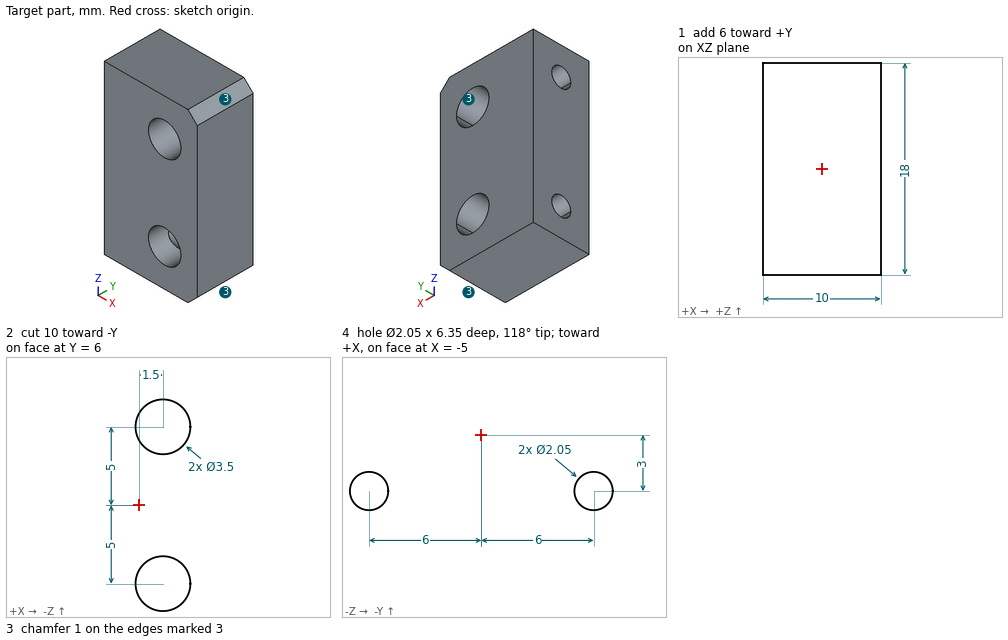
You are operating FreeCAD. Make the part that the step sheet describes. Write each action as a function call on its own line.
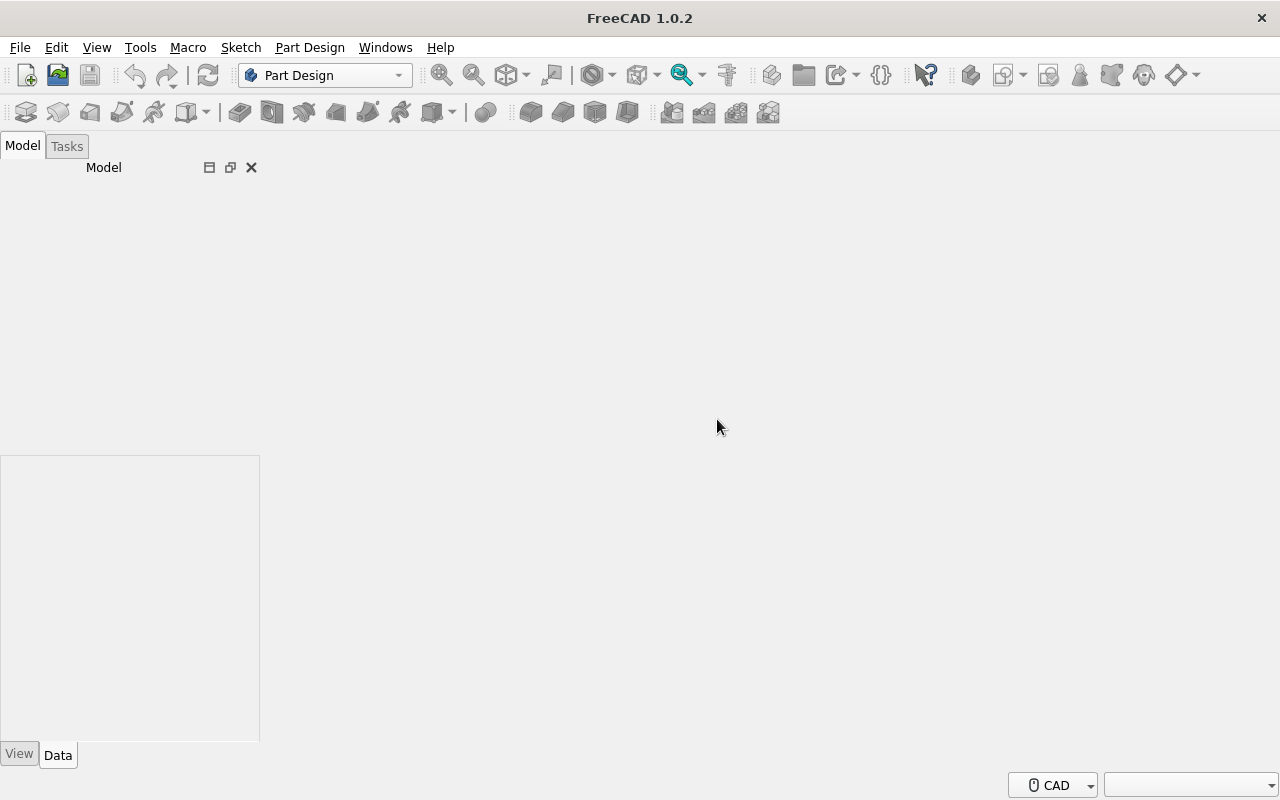
key(ctrl+n)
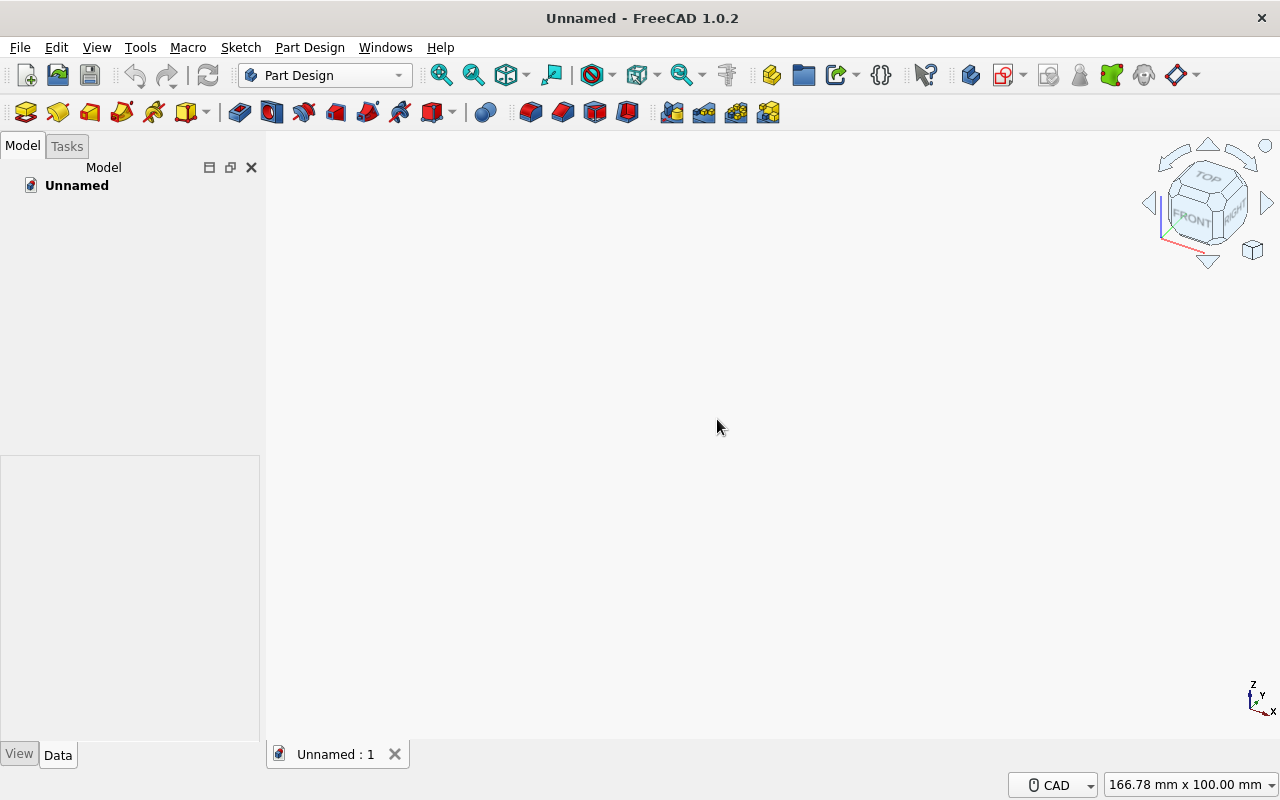
click(1004, 76)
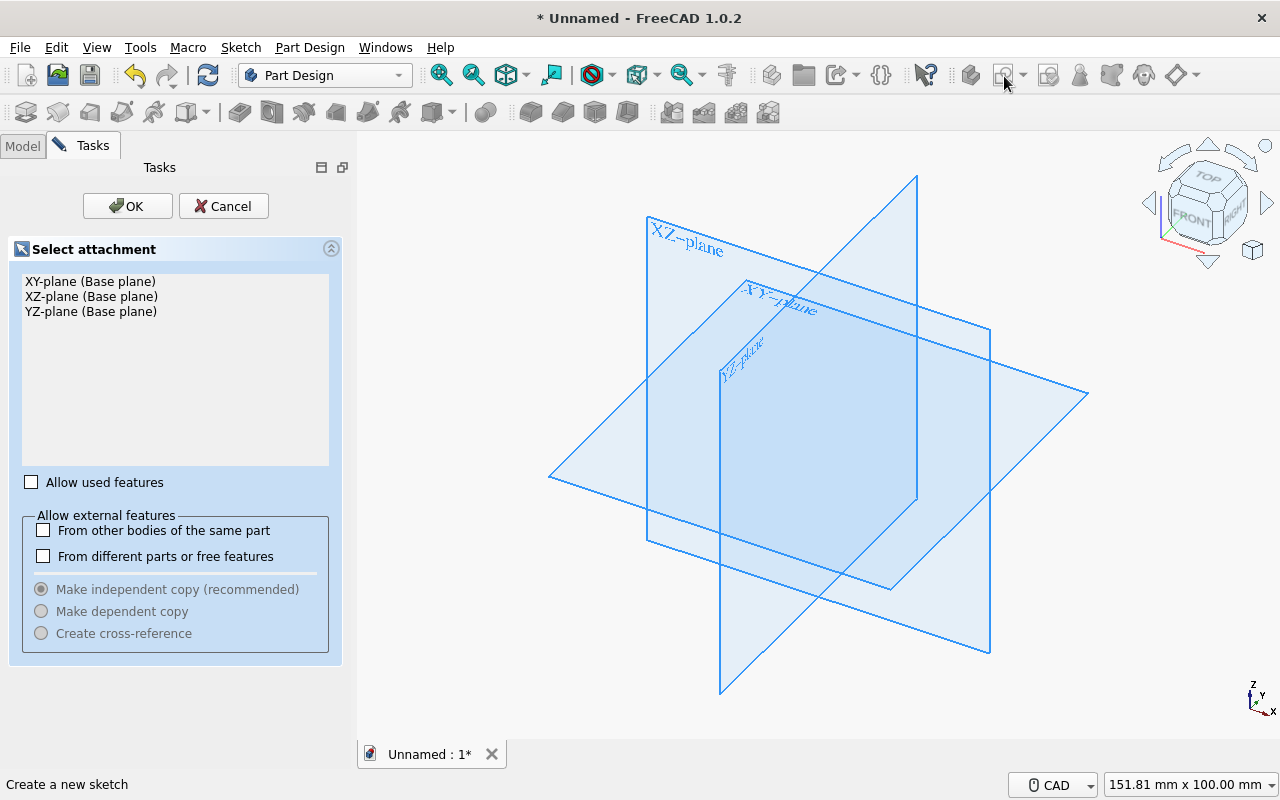
click(82, 296)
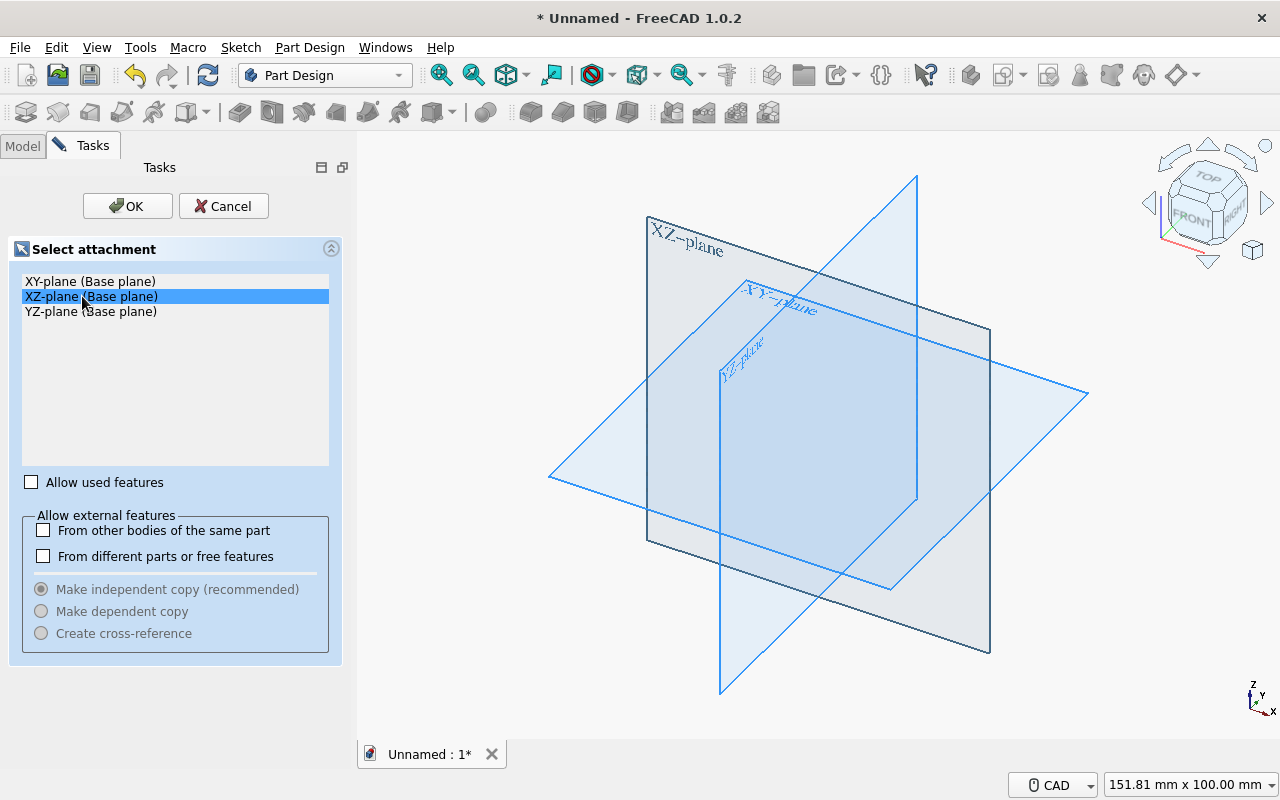
click(128, 206)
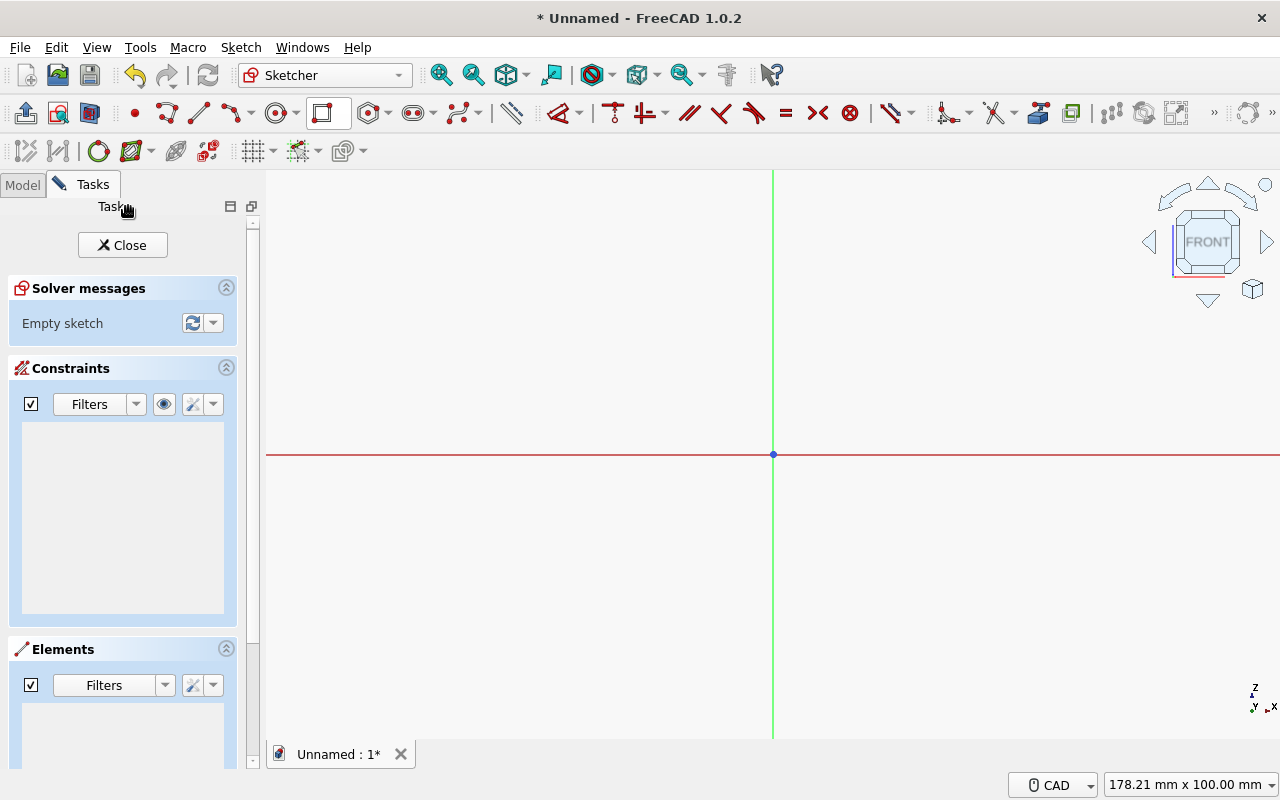
scroll(803, 455, up, 6)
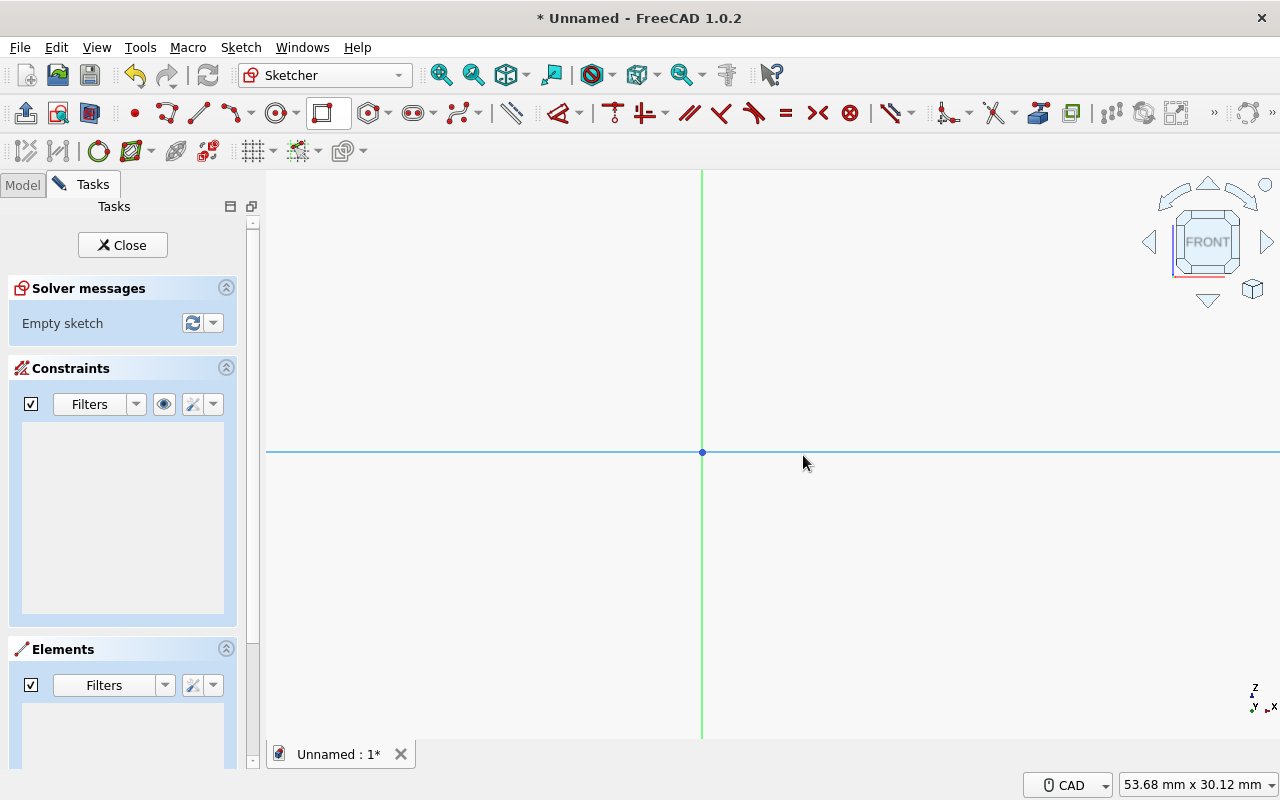
key(g)
key(v)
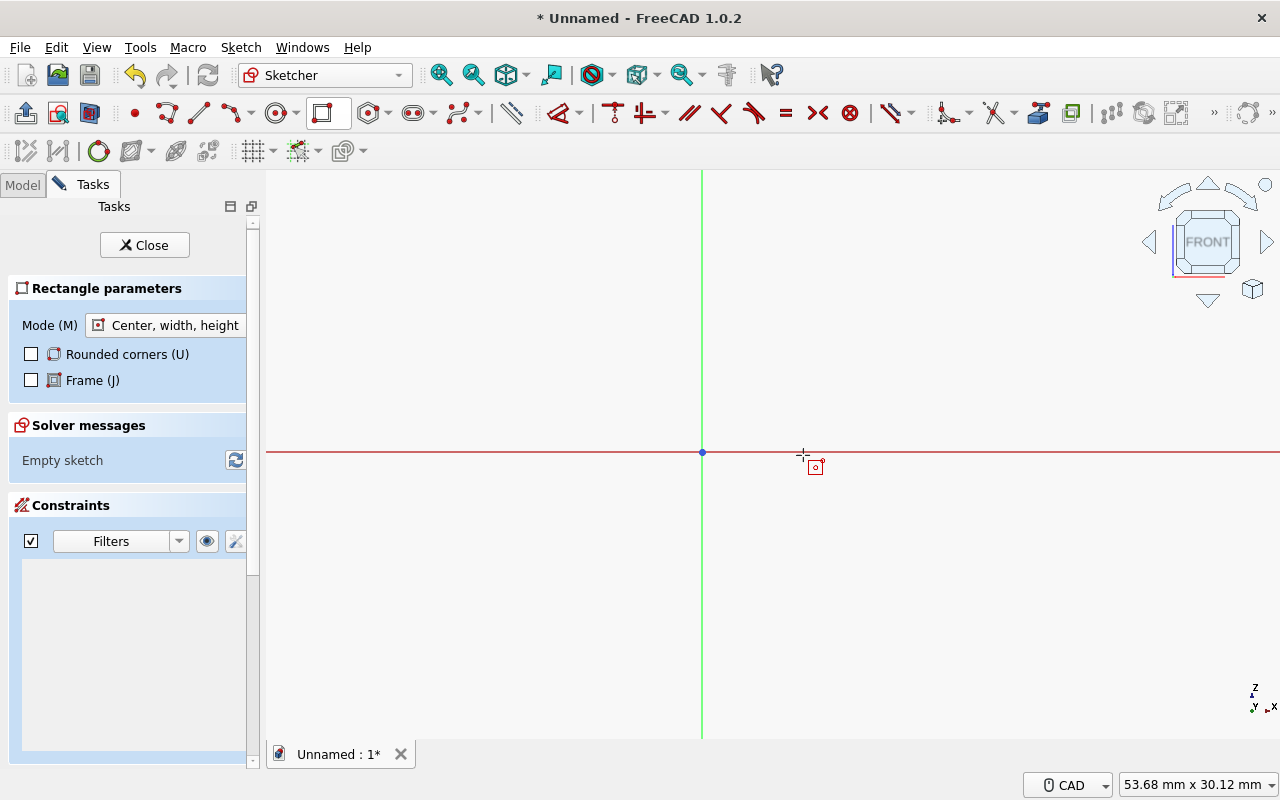
click(702, 452)
move(797, 282)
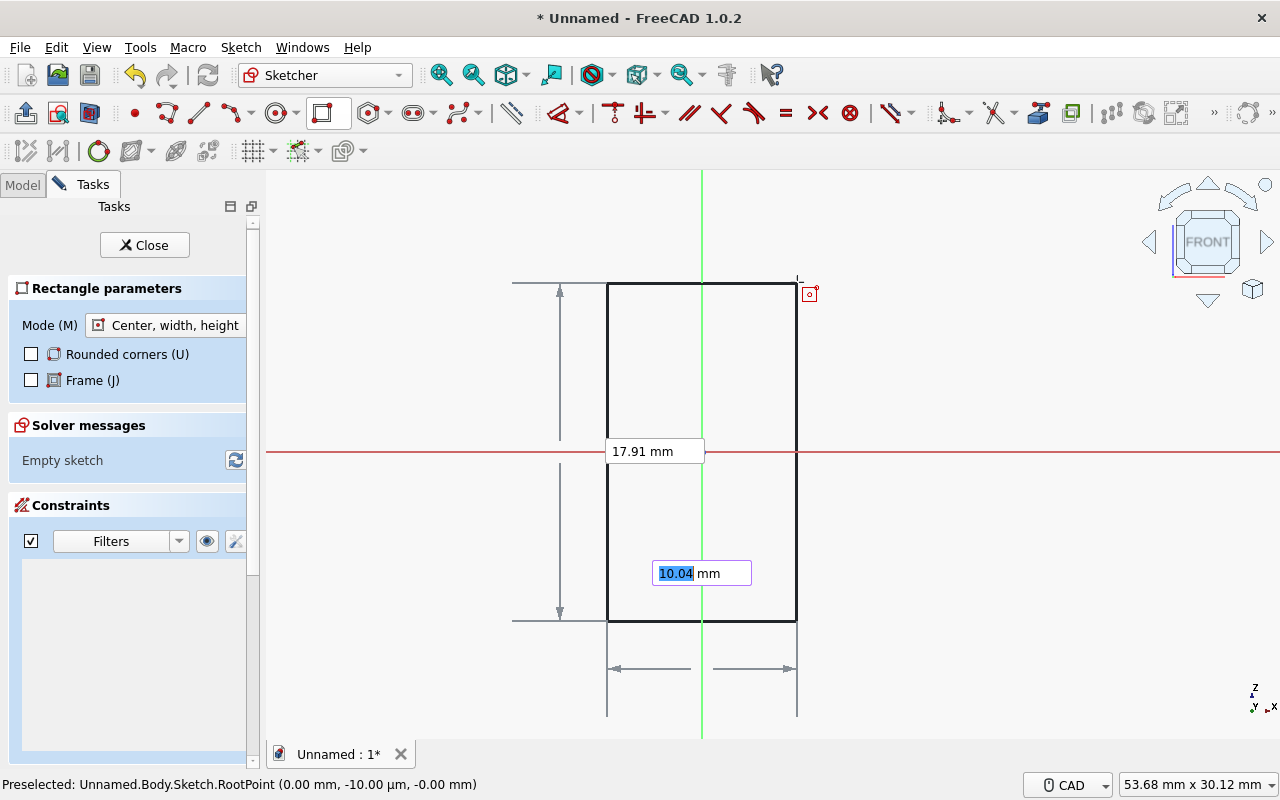
text(10)
key(Tab)
text(18)
key(Return)
key(Escape)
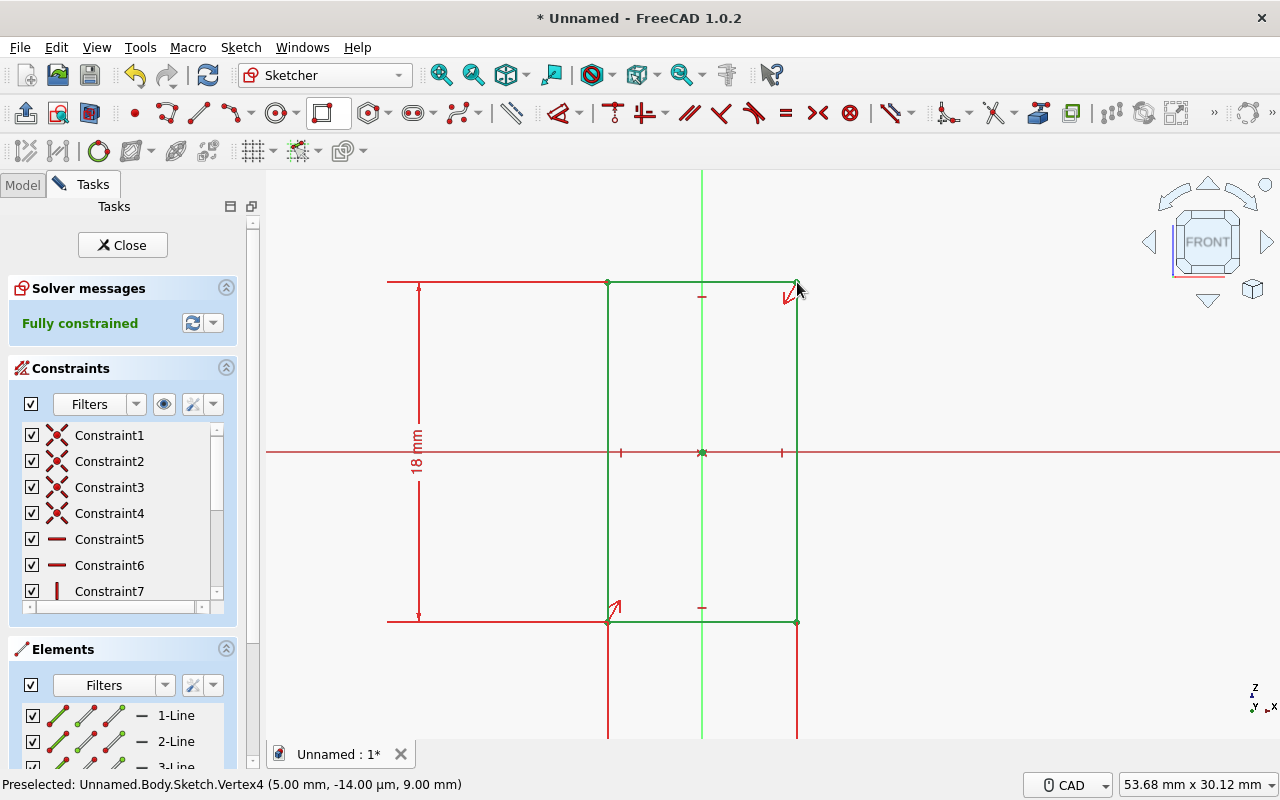
click(123, 245)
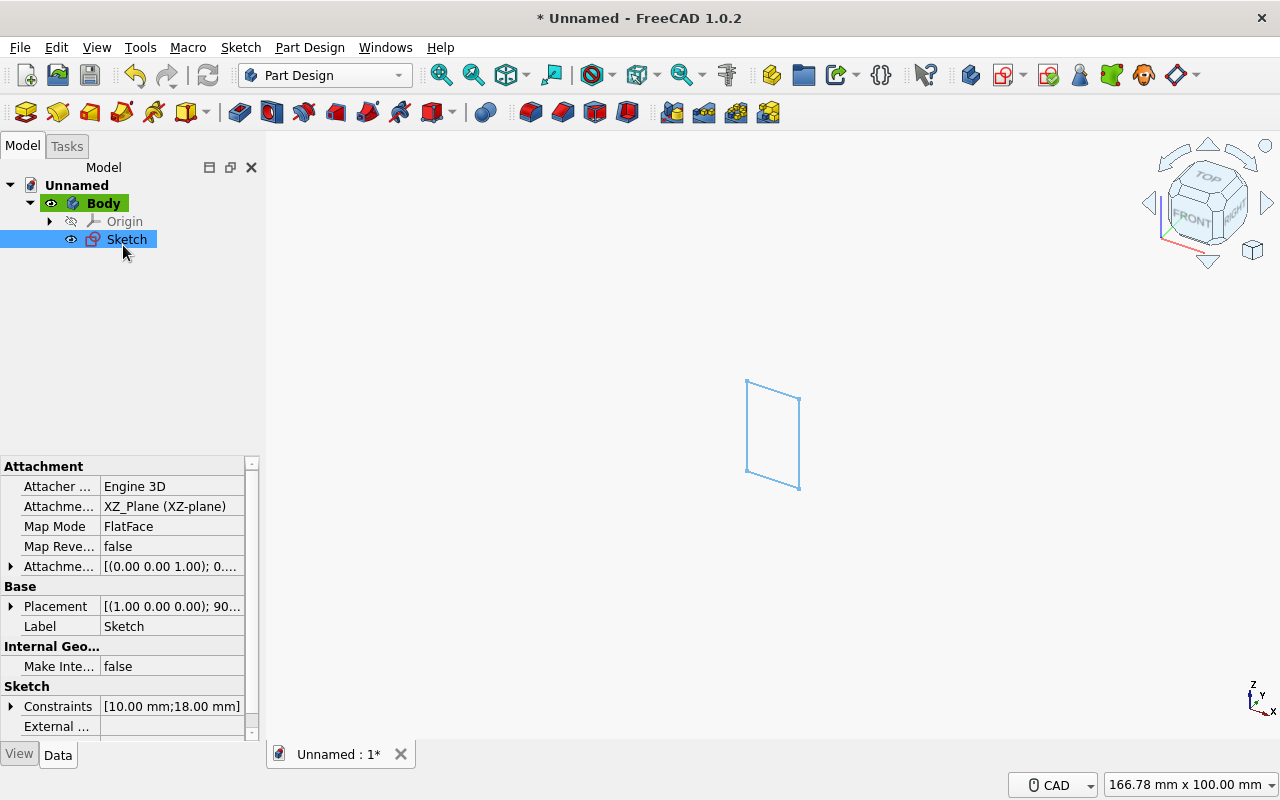
click(26, 112)